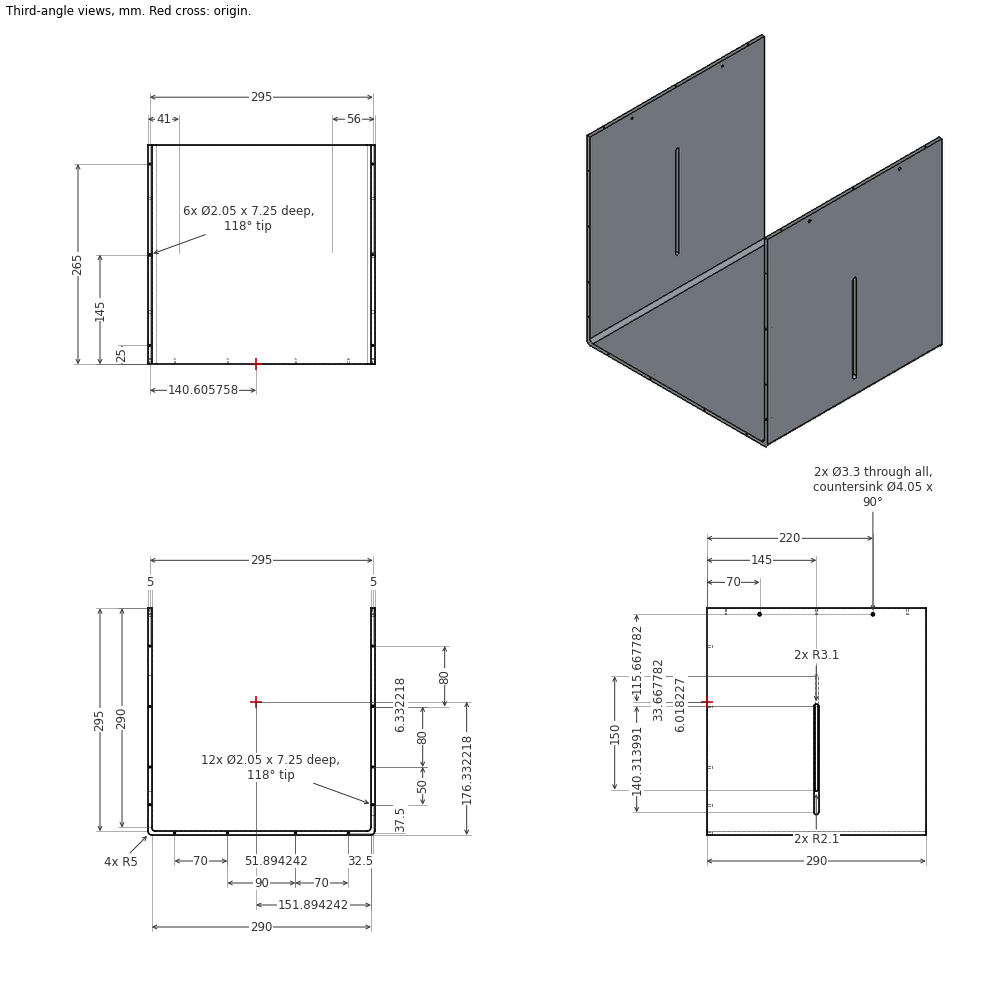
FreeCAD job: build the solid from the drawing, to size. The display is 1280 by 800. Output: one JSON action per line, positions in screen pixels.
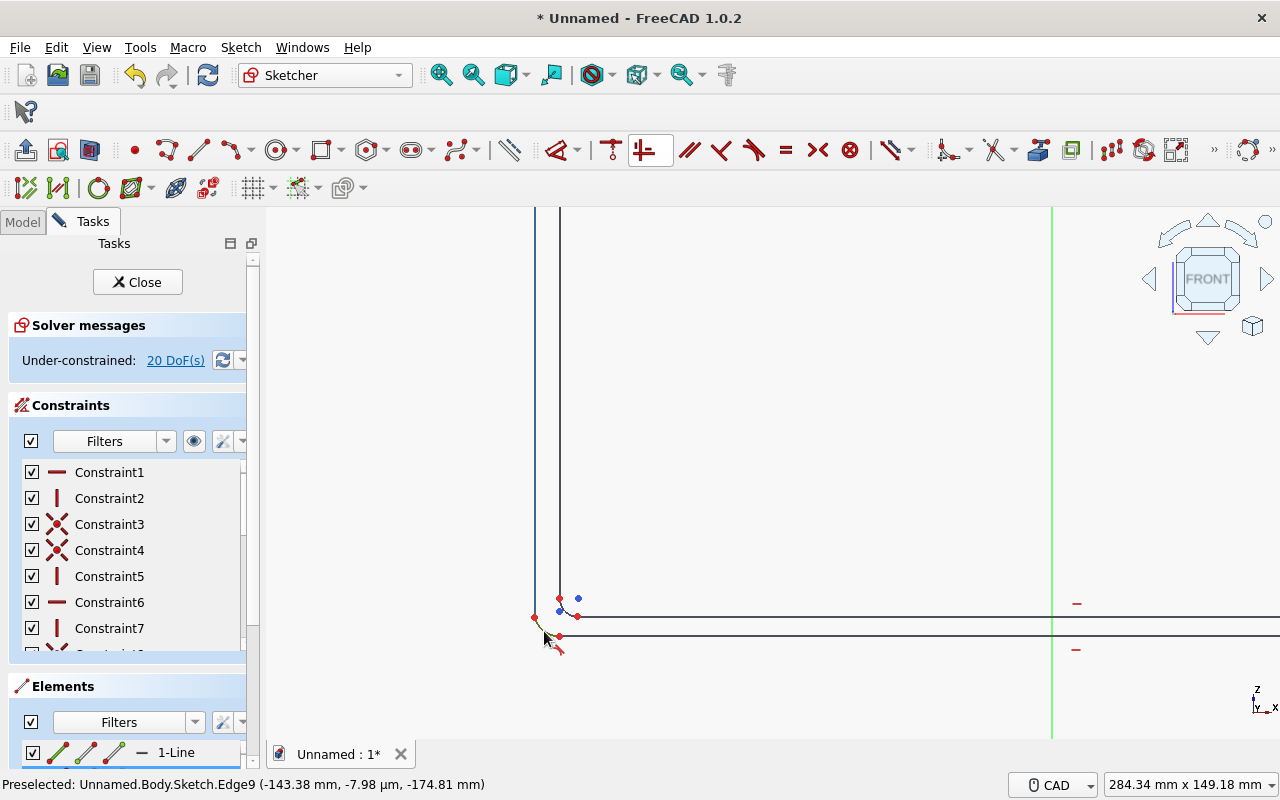
{"action": "left_click", "coordinate": [754, 150]}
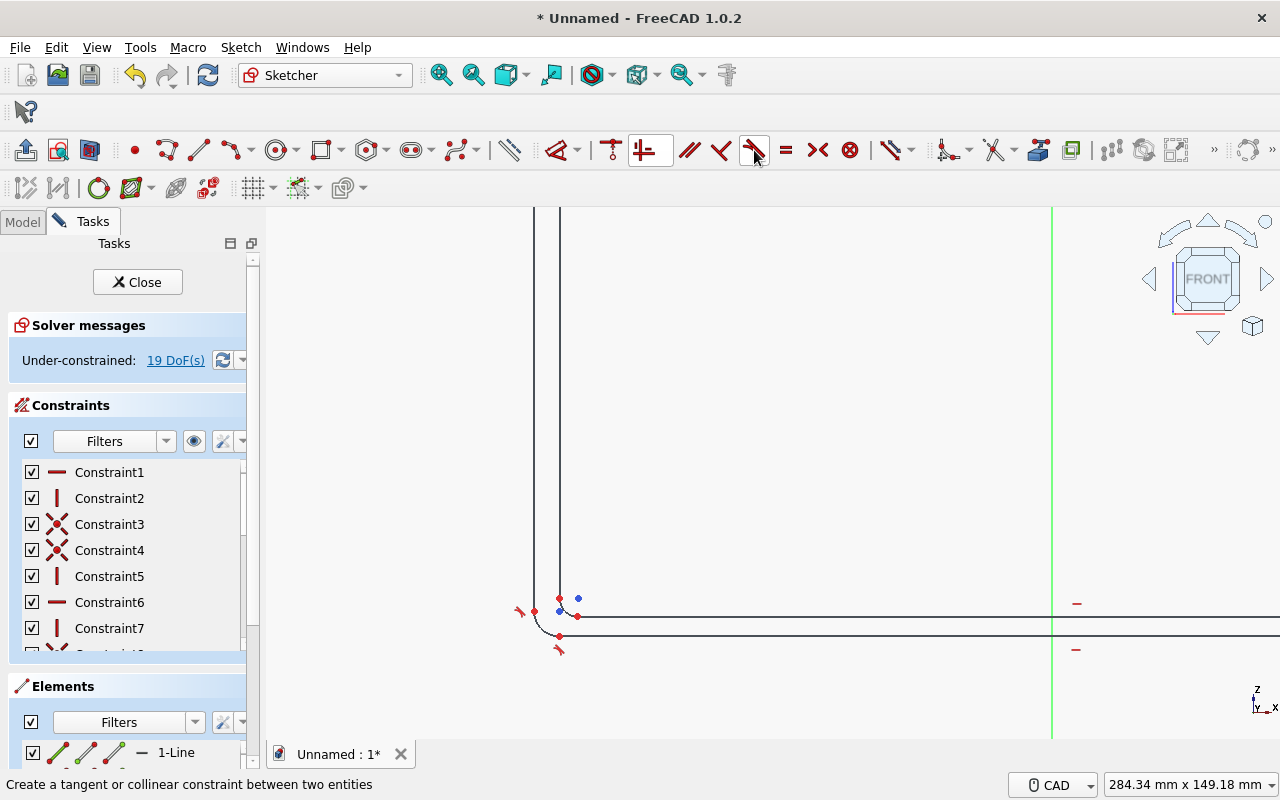
{"action": "left_click", "coordinate": [560, 289]}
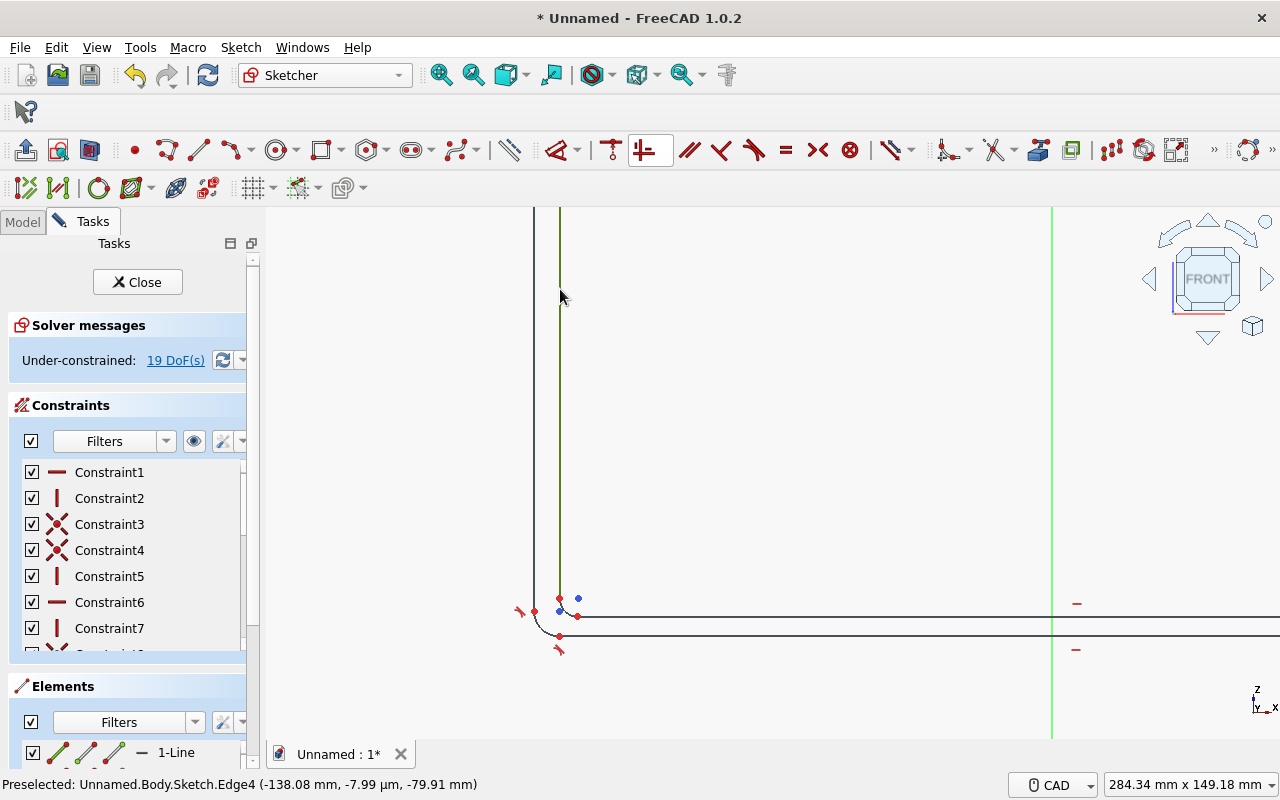
{"action": "left_click", "coordinate": [565, 611]}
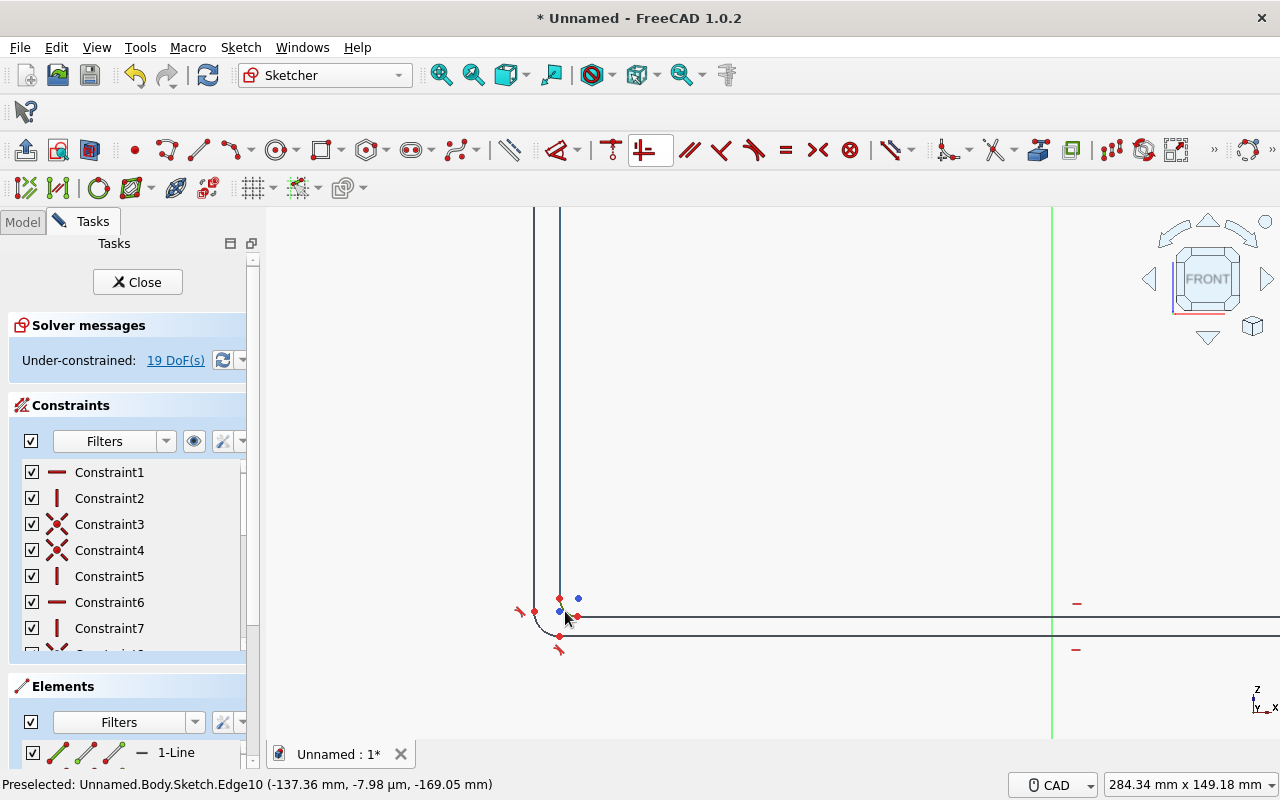
{"action": "left_click", "coordinate": [754, 150]}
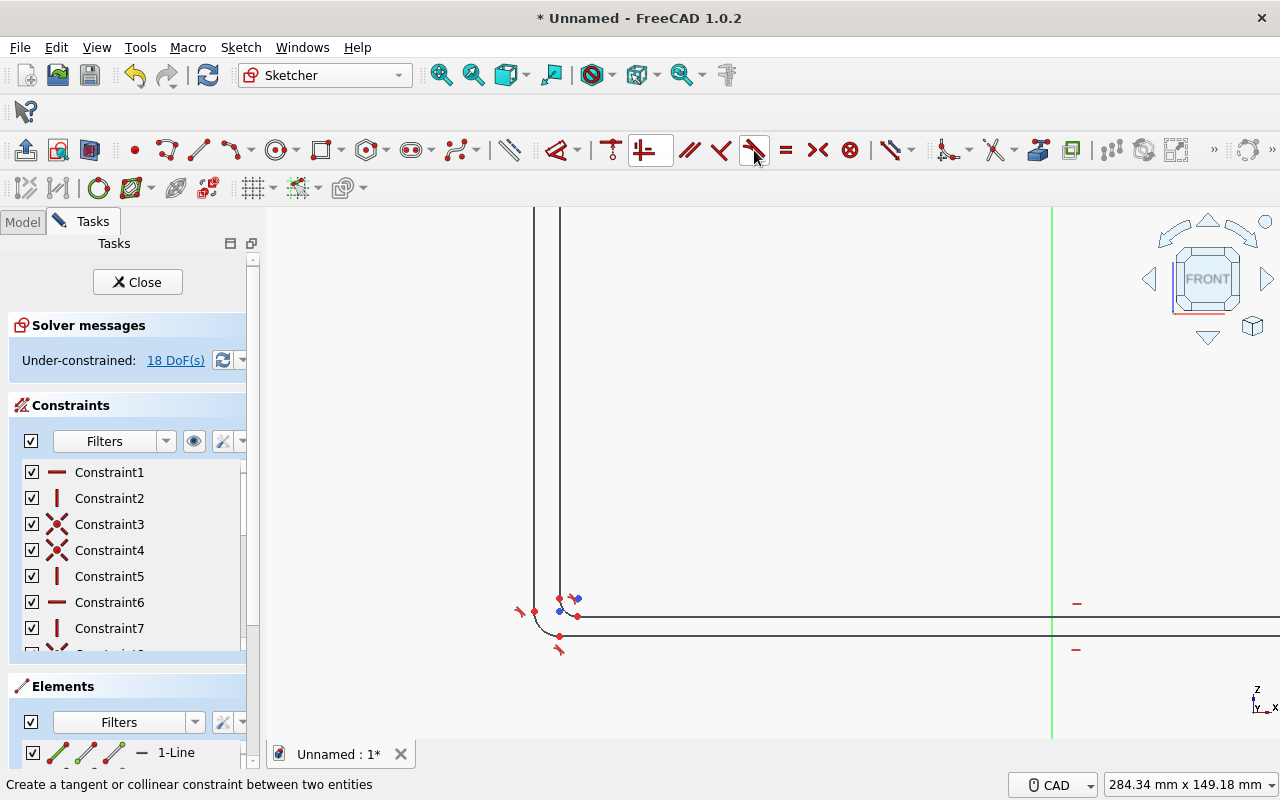
{"action": "left_click", "coordinate": [877, 617]}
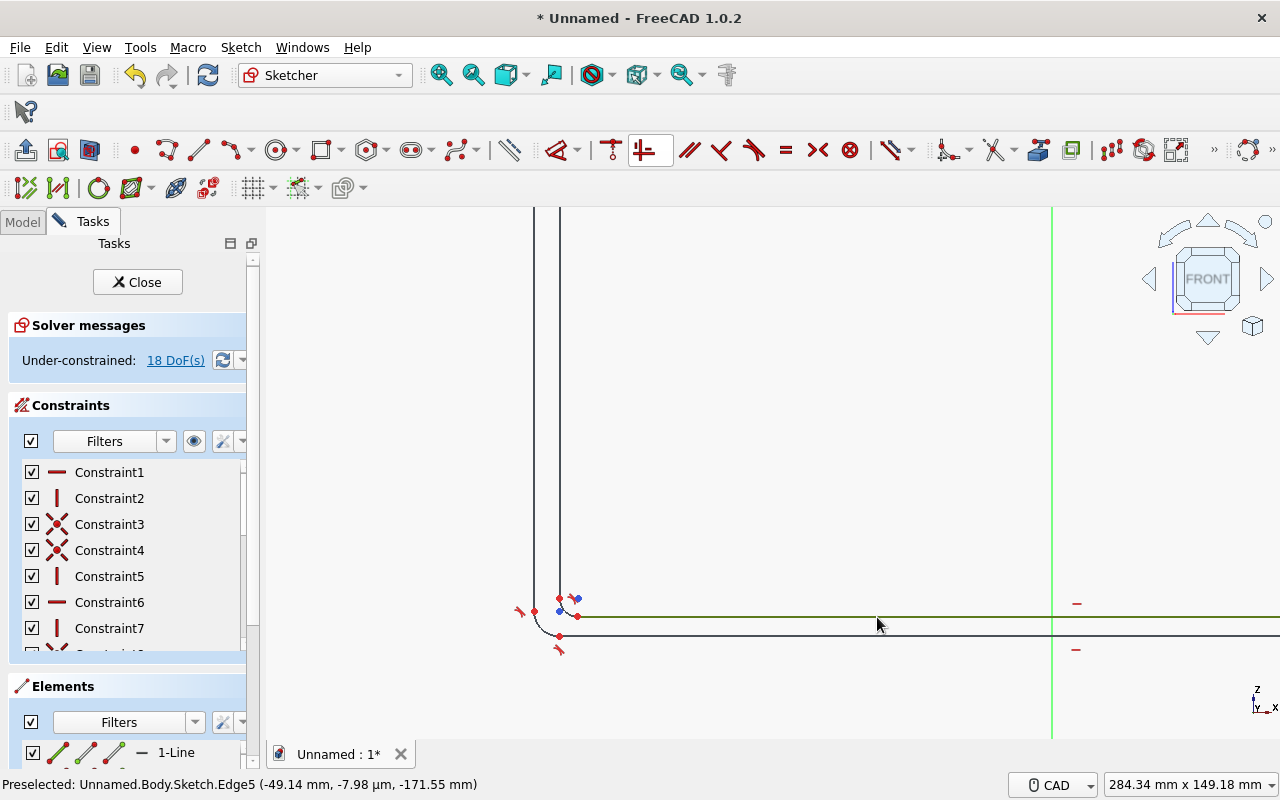
{"action": "left_click", "coordinate": [565, 611]}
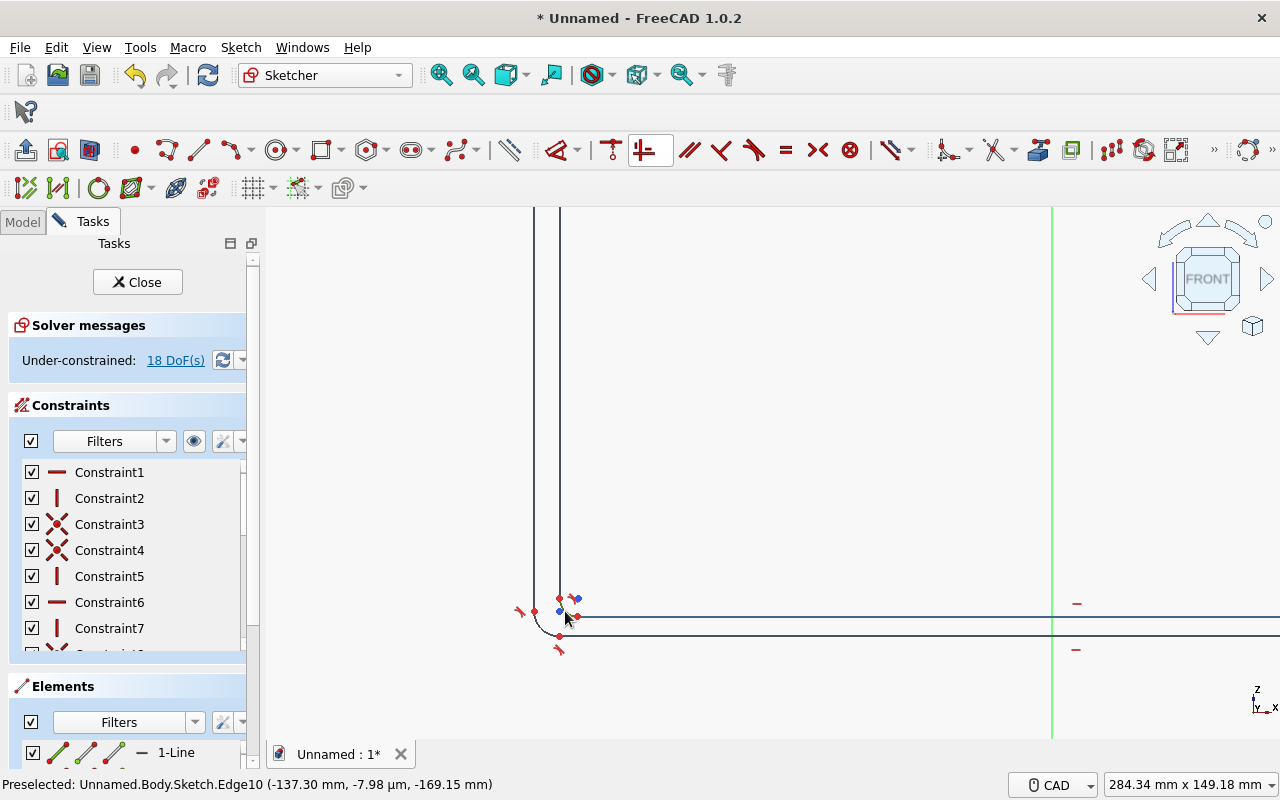
{"action": "left_click", "coordinate": [754, 150]}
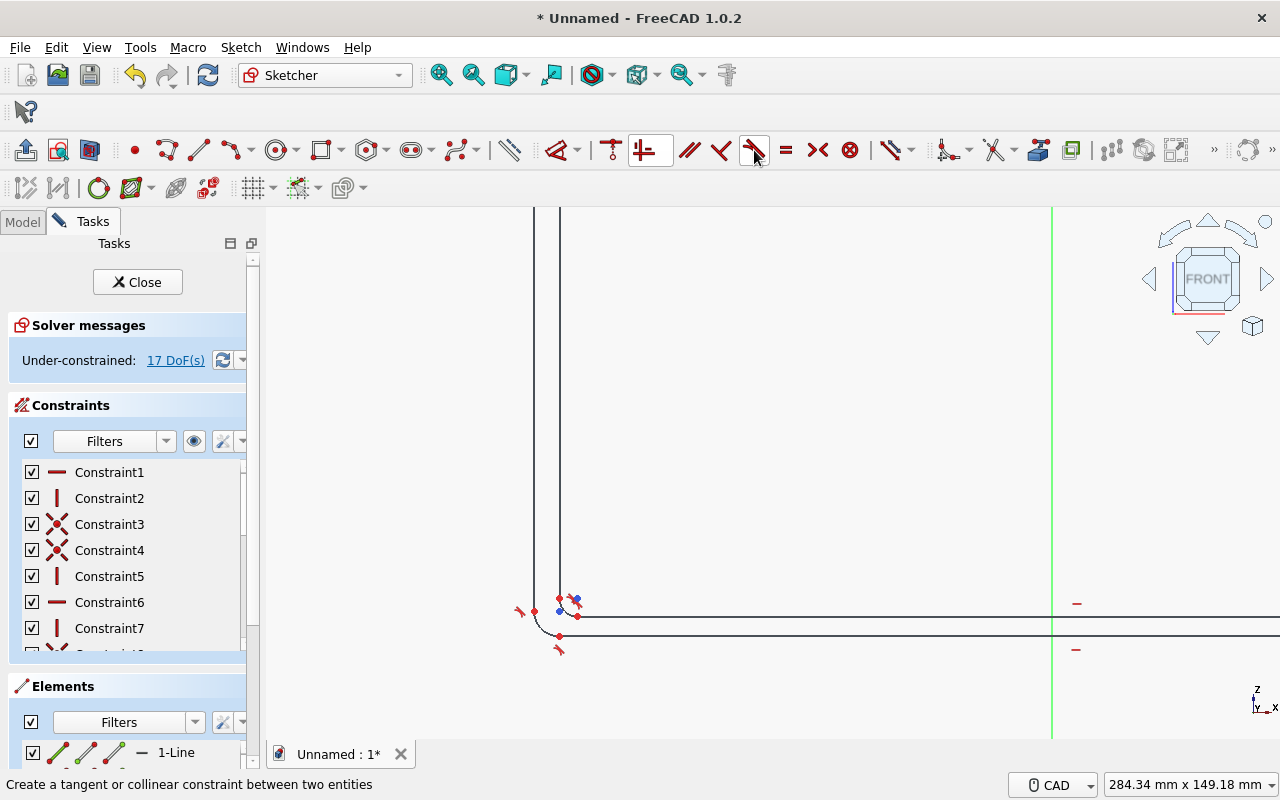
{"action": "left_click", "coordinate": [877, 617]}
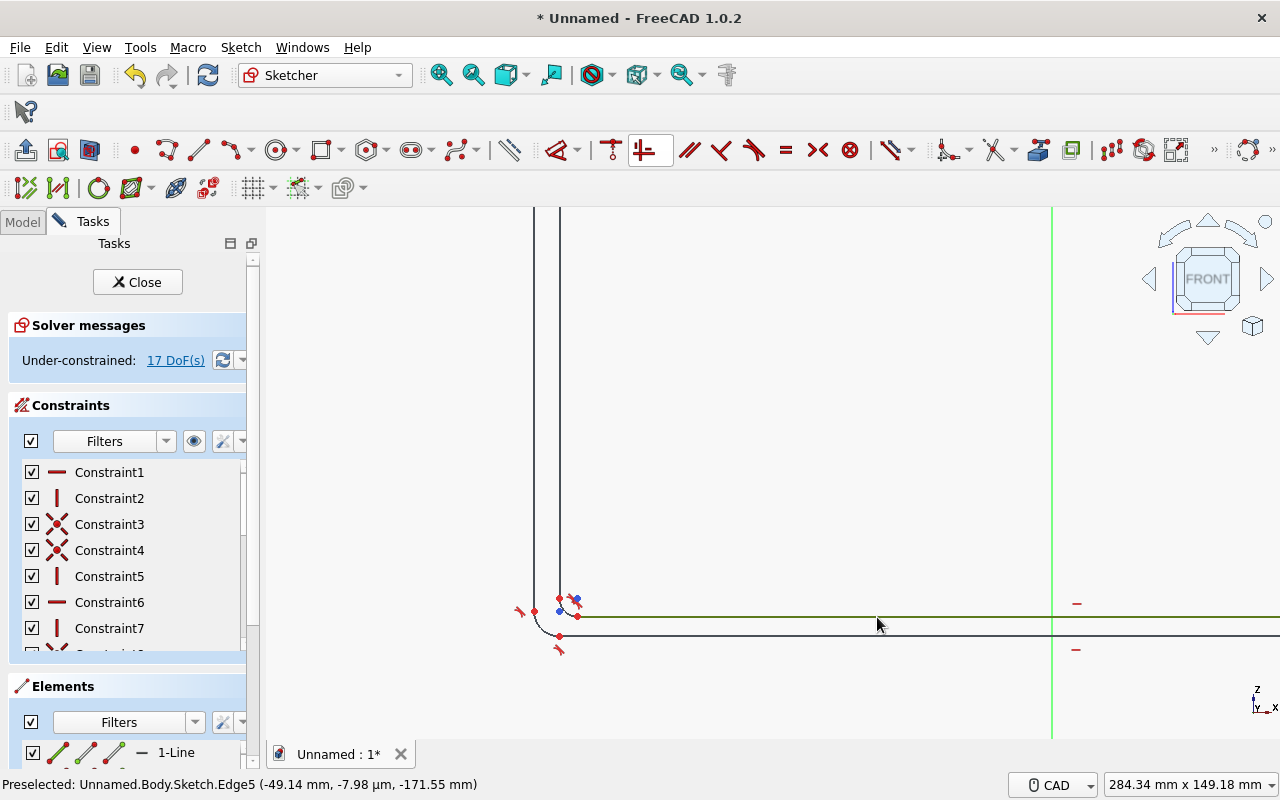
{"action": "scroll", "coordinate": [544, 634], "scroll_direction": "down", "scroll_amount": 6}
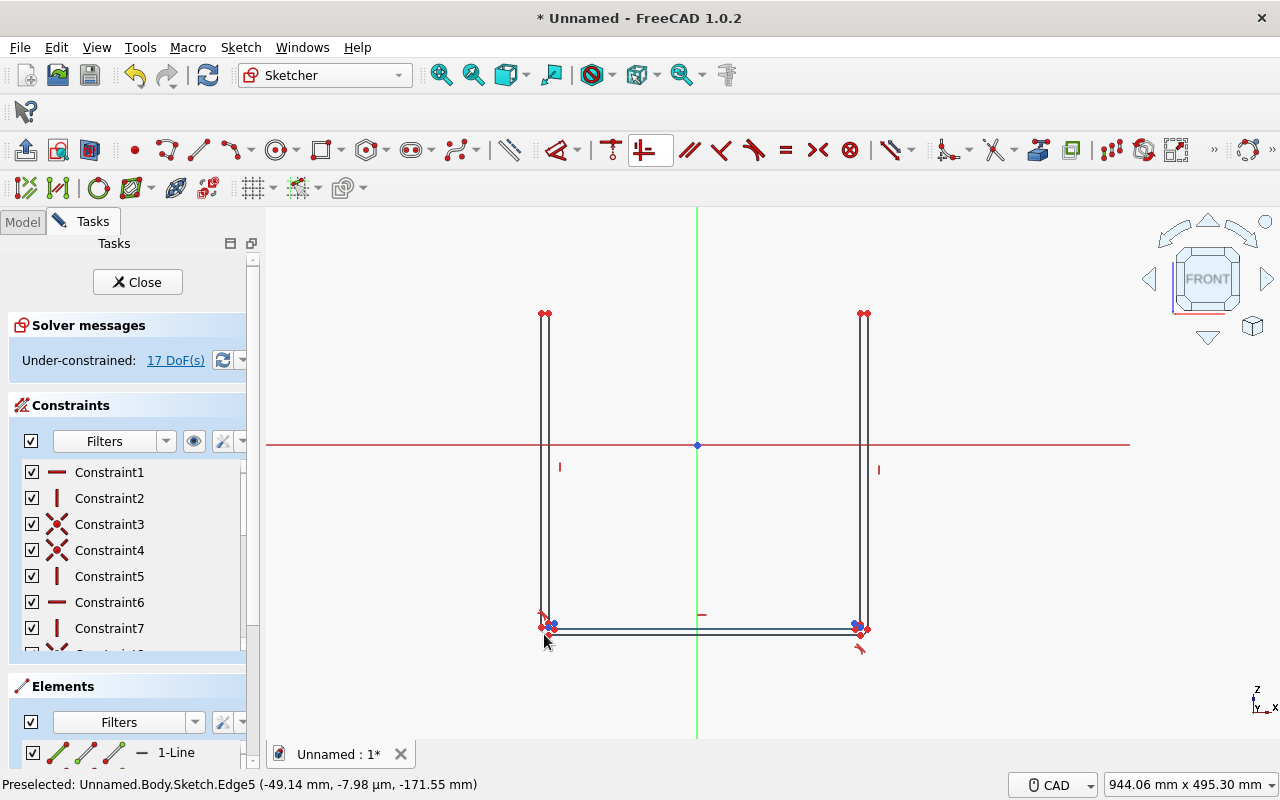
{"action": "scroll", "coordinate": [859, 628], "scroll_direction": "up", "scroll_amount": 7}